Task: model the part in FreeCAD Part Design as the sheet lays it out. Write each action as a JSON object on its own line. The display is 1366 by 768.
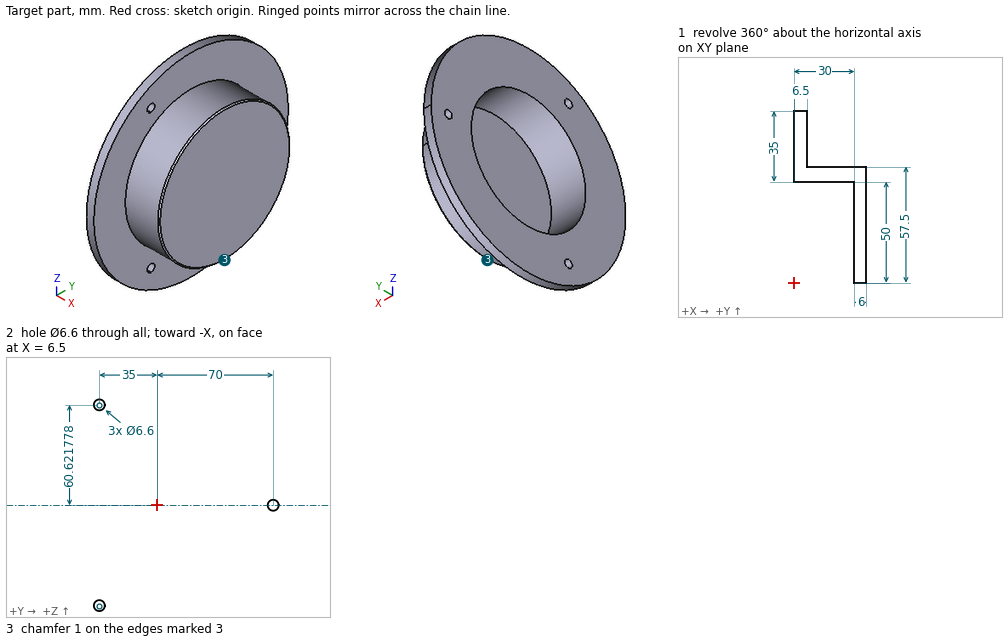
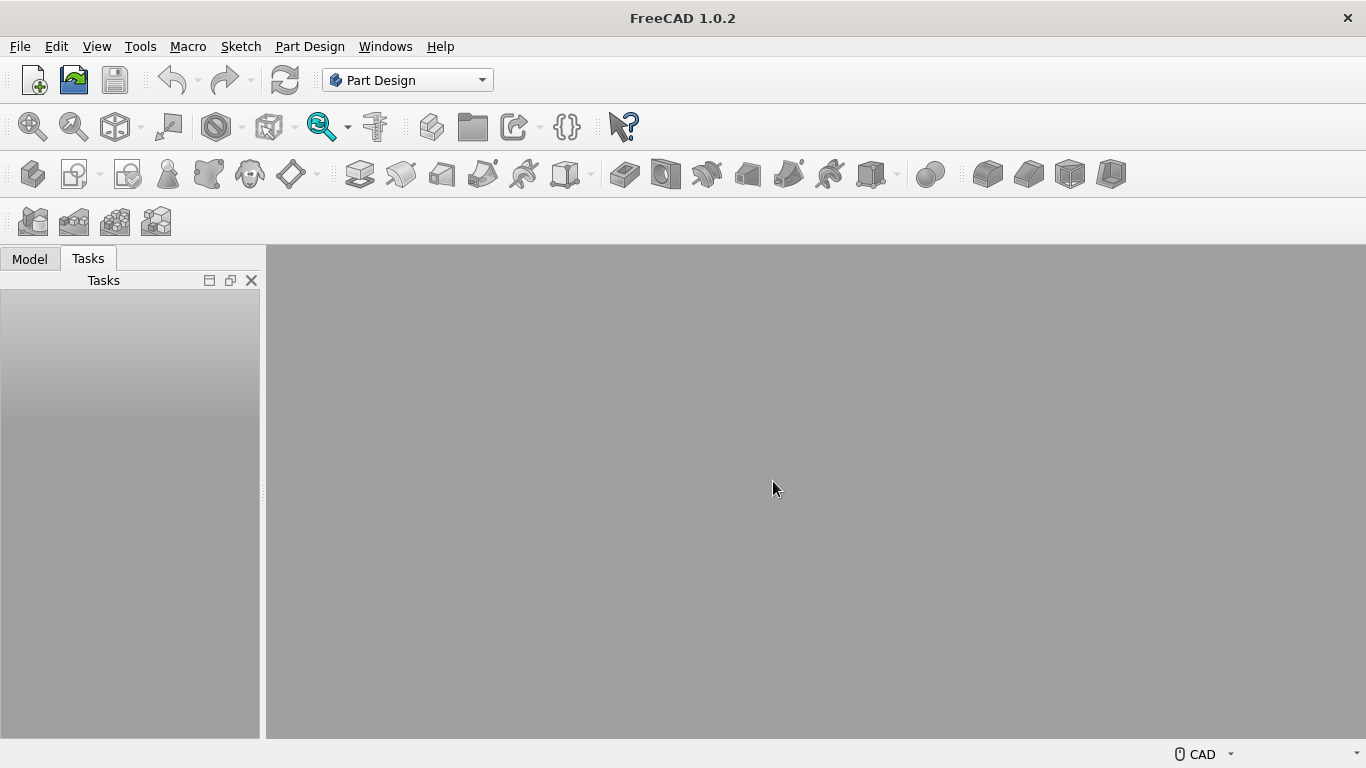
{"action": "left_click", "coordinate": [33, 80]}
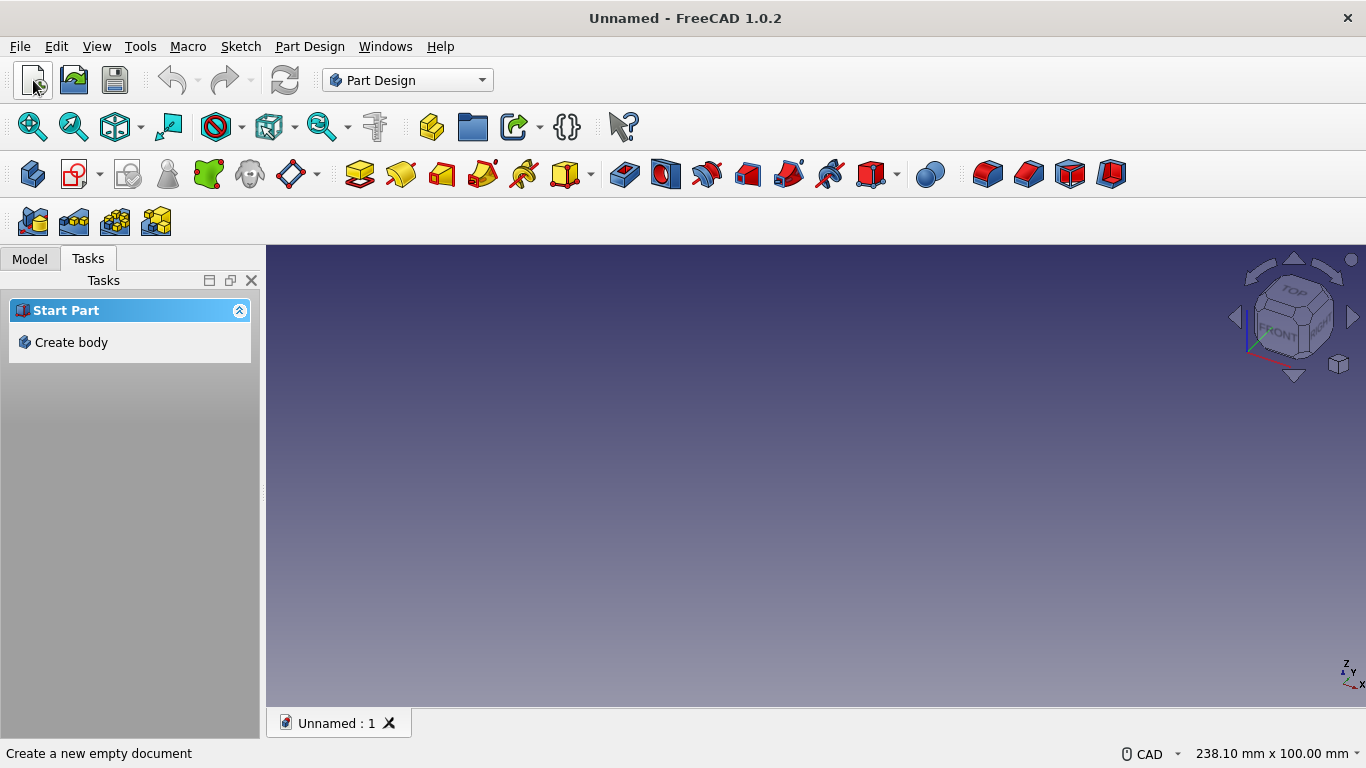
{"action": "left_click", "coordinate": [74, 174]}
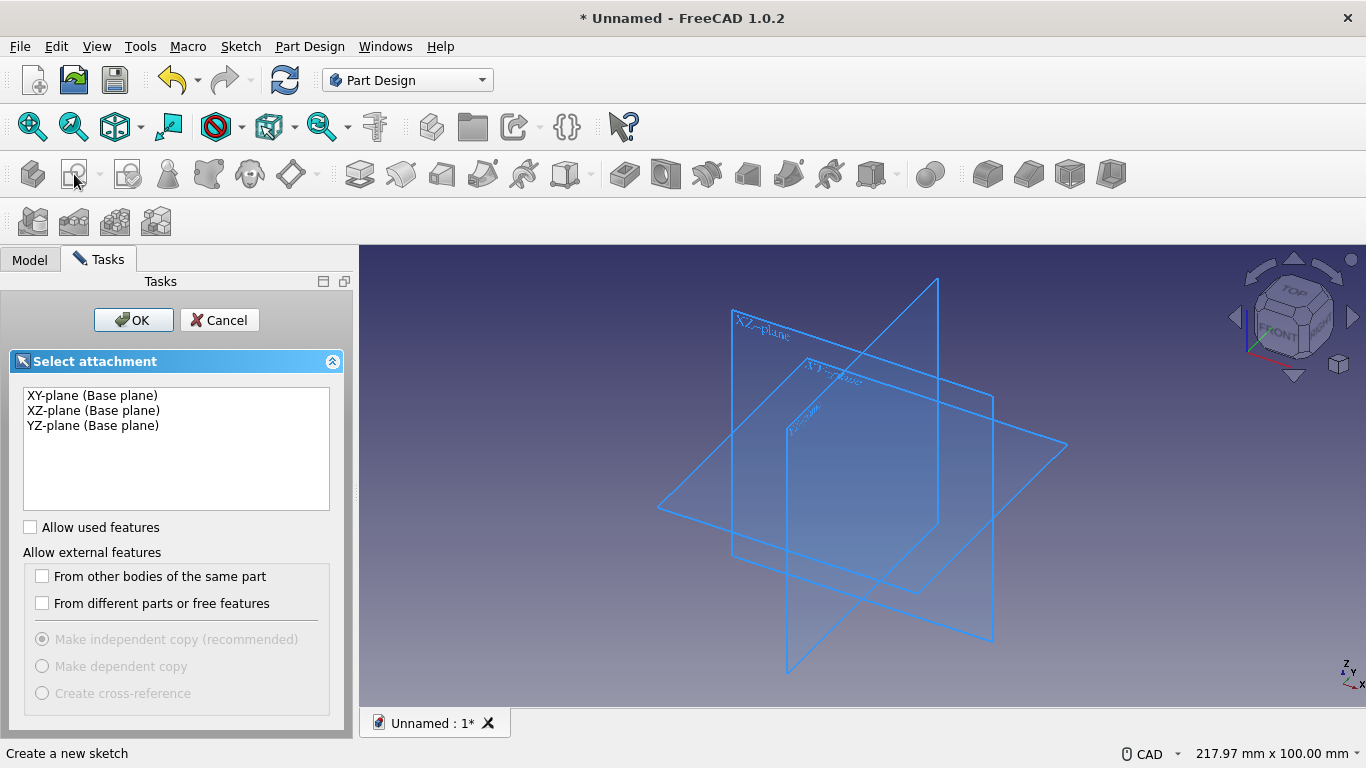
{"action": "left_click", "coordinate": [84, 396]}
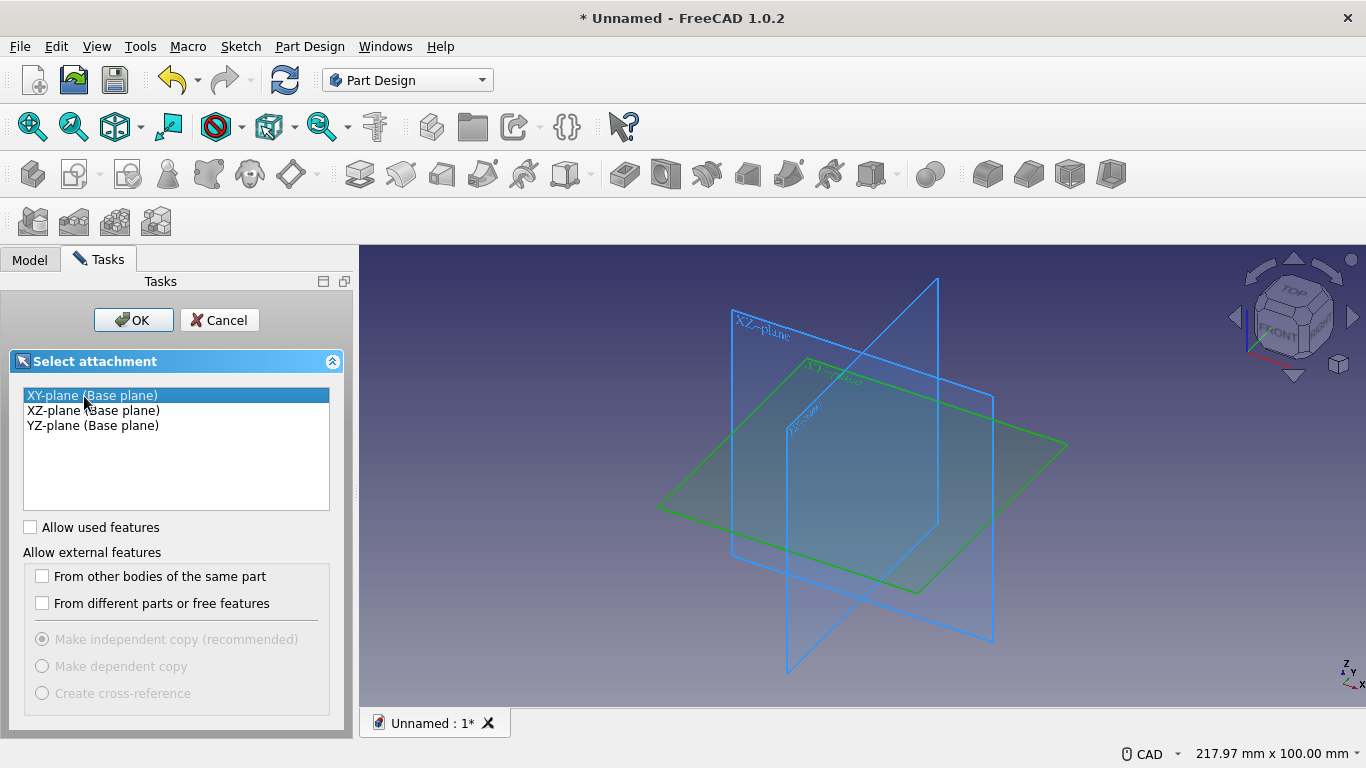
{"action": "left_click", "coordinate": [134, 320]}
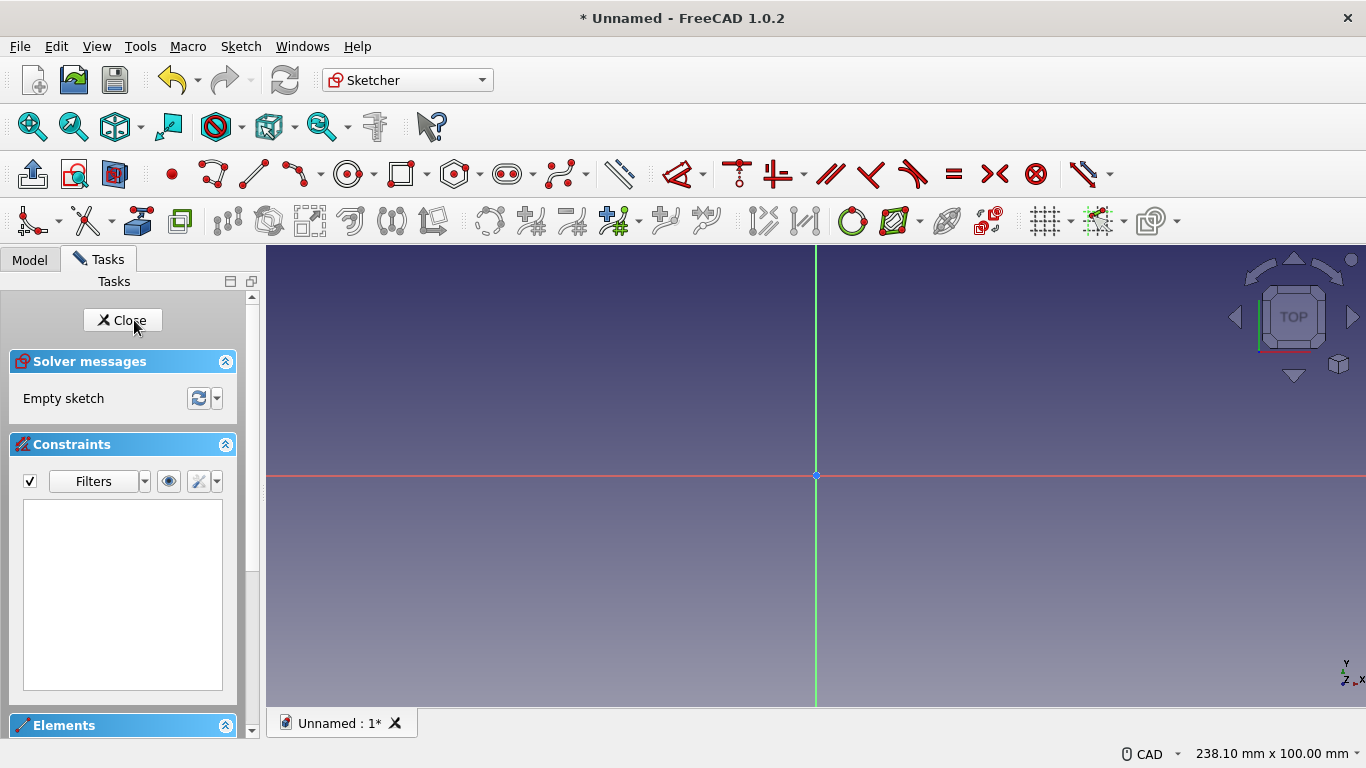
{"action": "scroll", "coordinate": [563, 679], "scroll_direction": "down", "scroll_amount": 3}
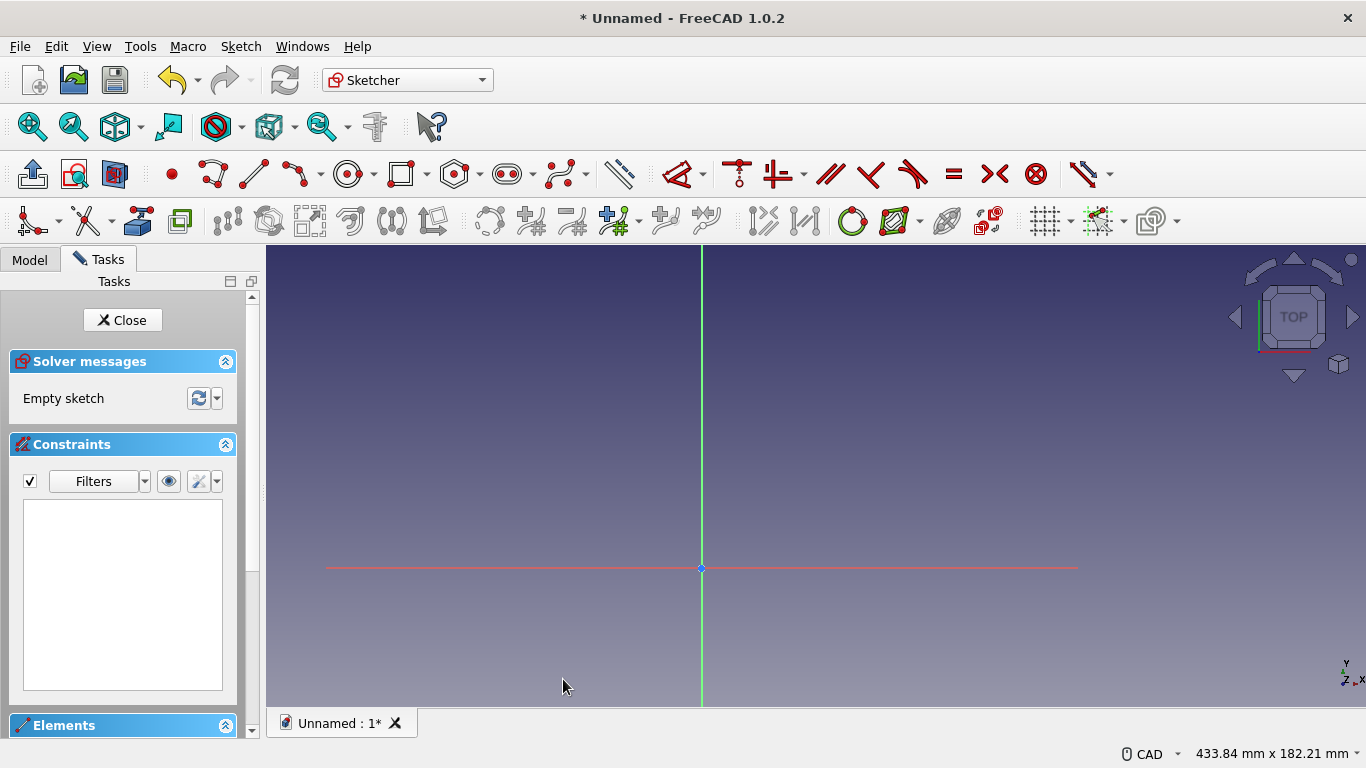
{"action": "left_click", "coordinate": [213, 174]}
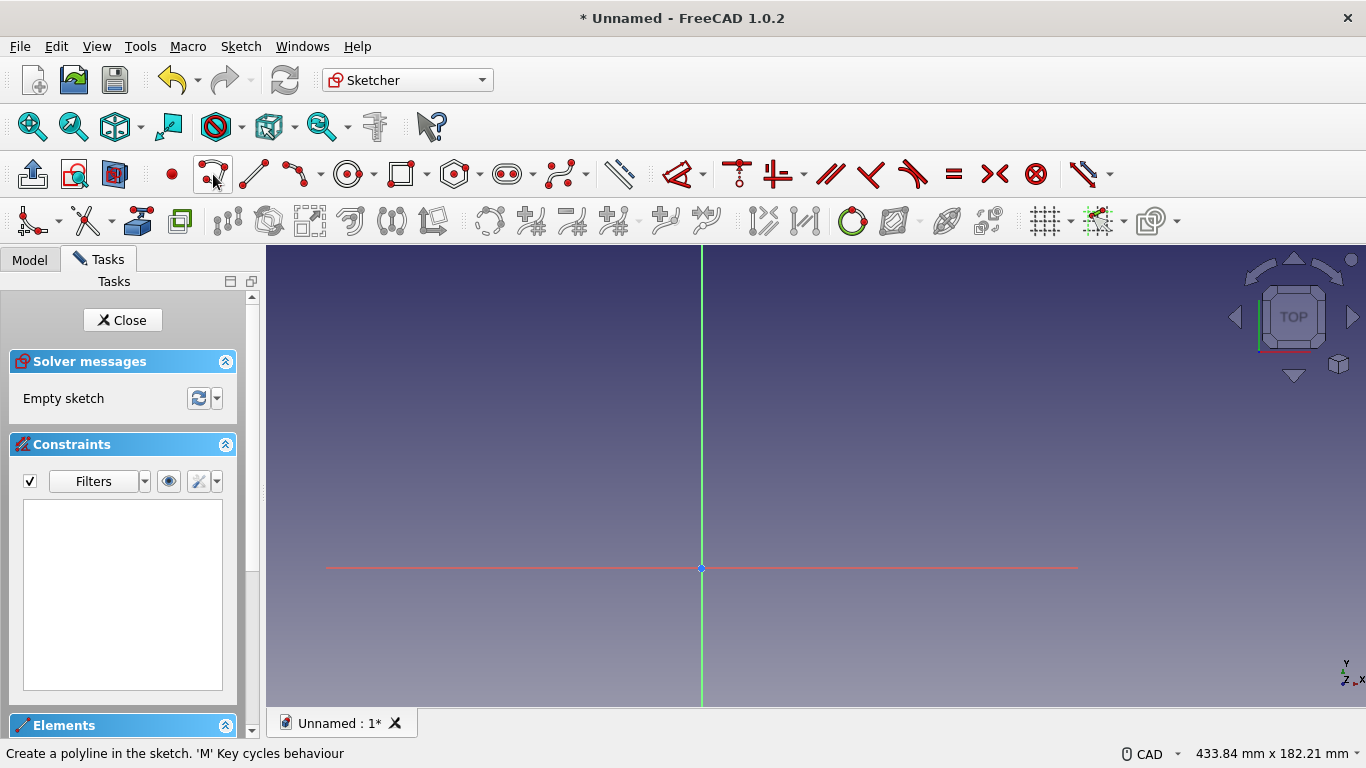
{"action": "left_click", "coordinate": [778, 568]}
{"action": "left_click", "coordinate": [793, 559]}
{"action": "left_click", "coordinate": [793, 422]}
{"action": "left_click", "coordinate": [718, 422]}
{"action": "left_click", "coordinate": [718, 352]}
{"action": "left_click", "coordinate": [702, 352]}
{"action": "left_click", "coordinate": [711, 441]}
{"action": "left_click", "coordinate": [778, 441]}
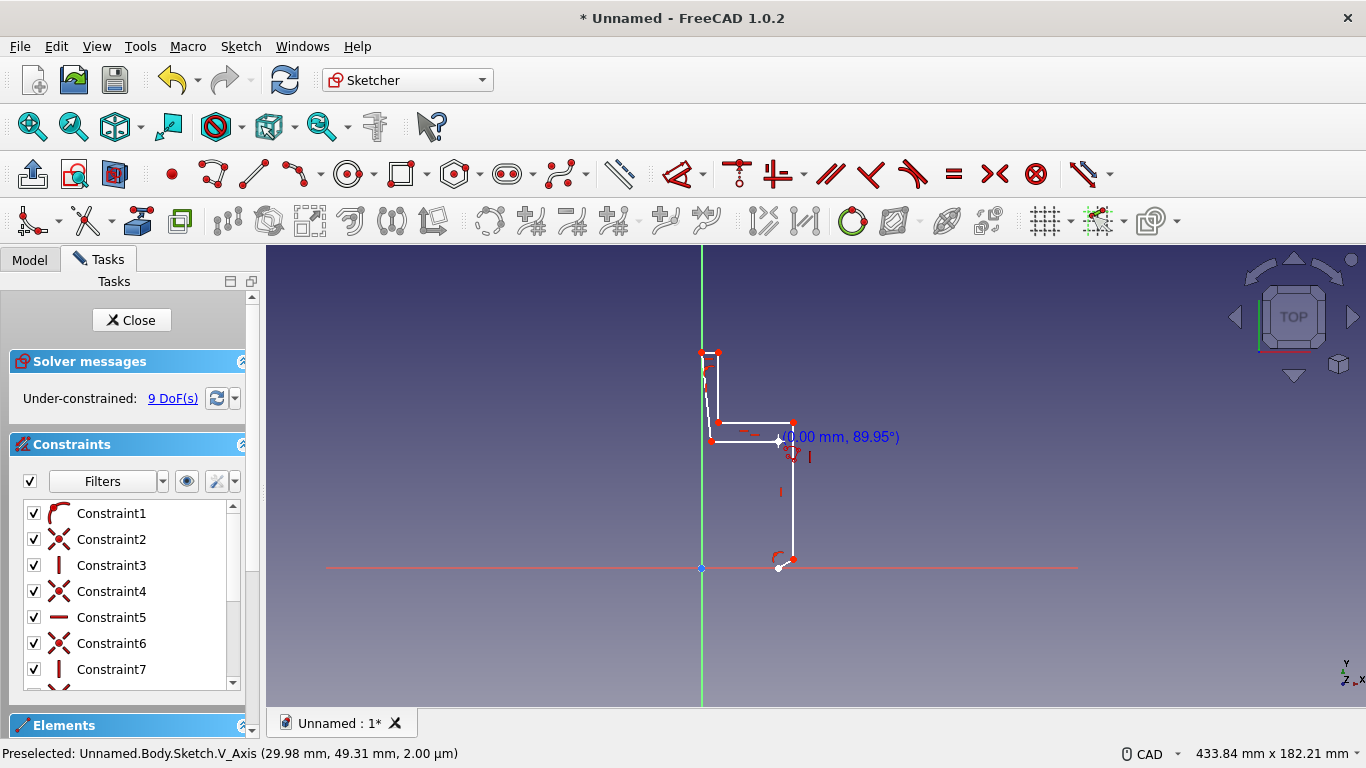
{"action": "scroll", "coordinate": [778, 568], "scroll_direction": "up", "scroll_amount": 4}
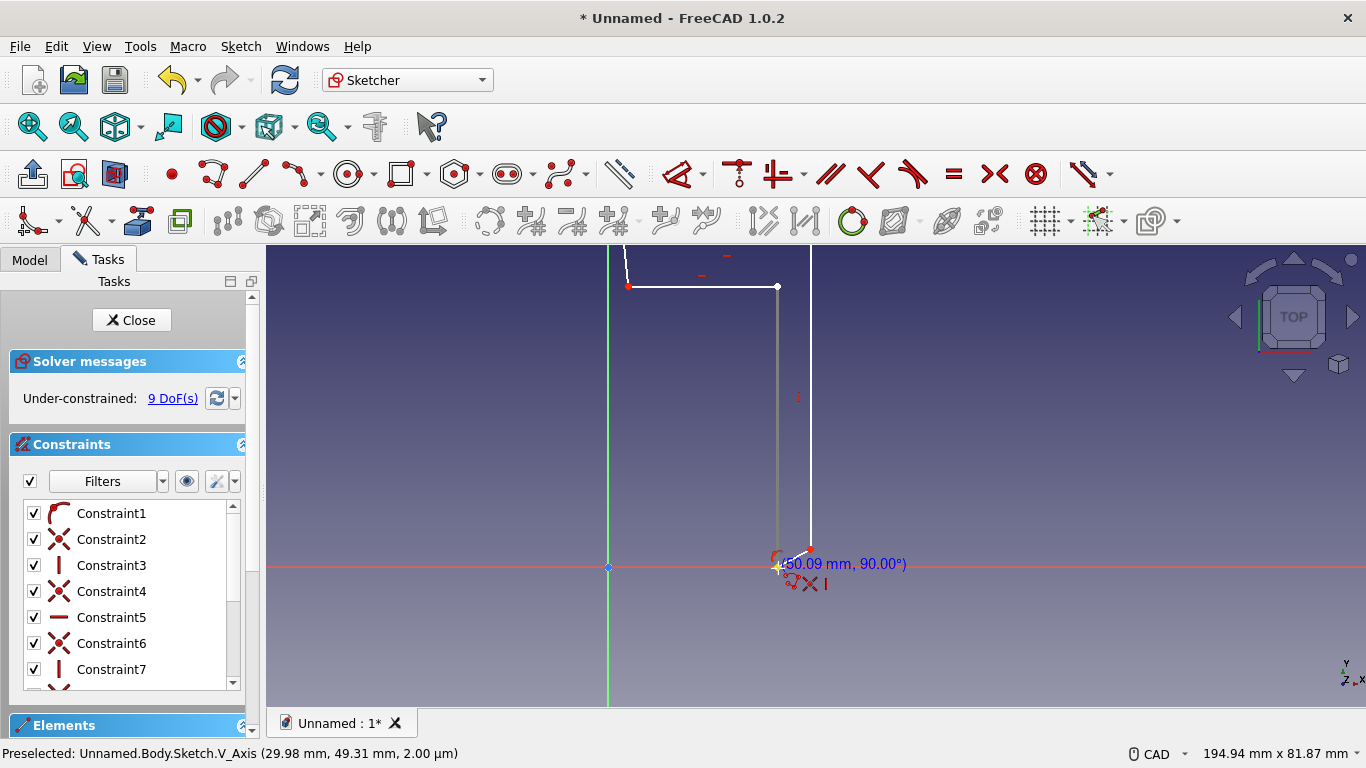
{"action": "left_click", "coordinate": [777, 567]}
{"action": "key", "text": "Escape"}
{"action": "key", "text": "Escape"}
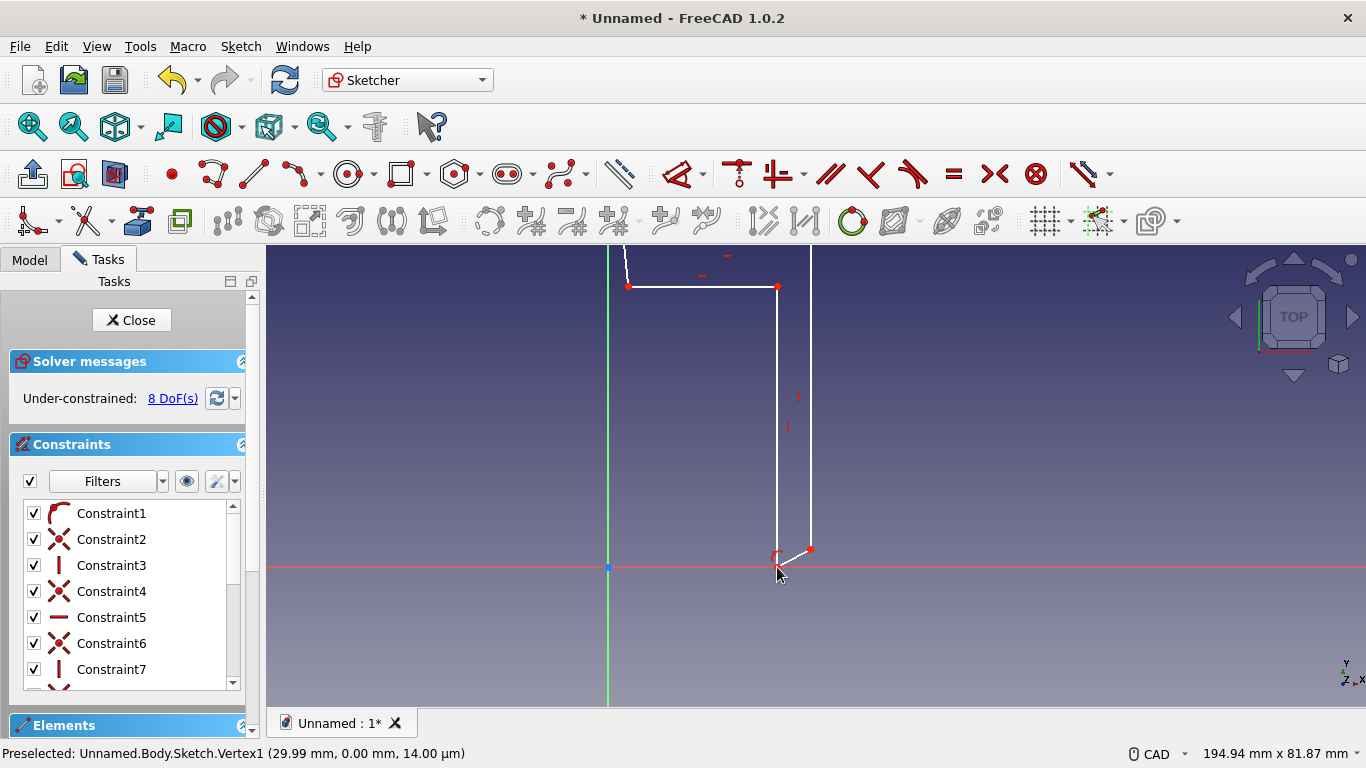
{"action": "left_click", "coordinate": [801, 555]}